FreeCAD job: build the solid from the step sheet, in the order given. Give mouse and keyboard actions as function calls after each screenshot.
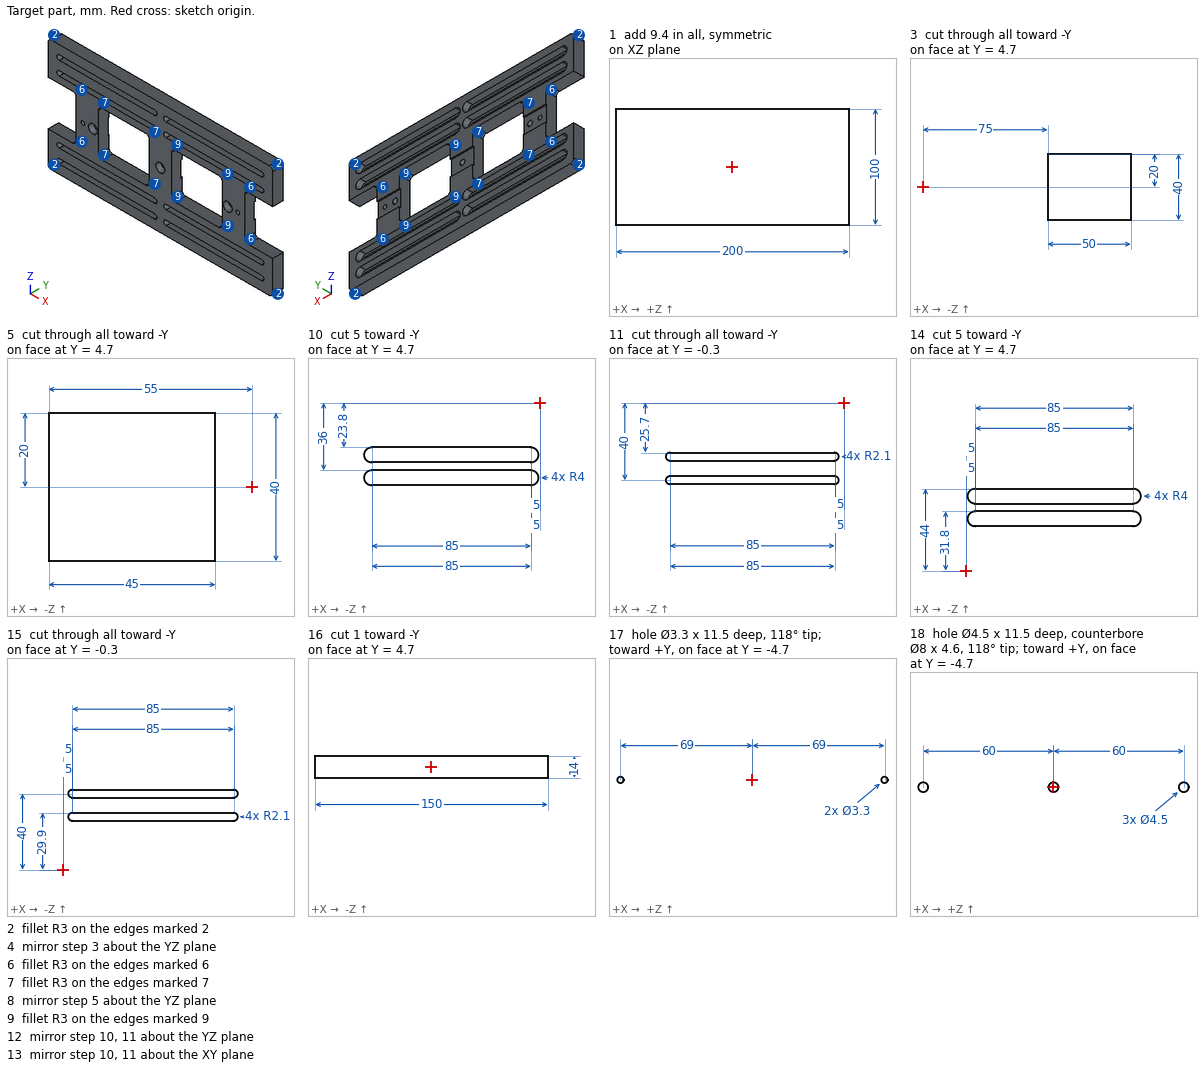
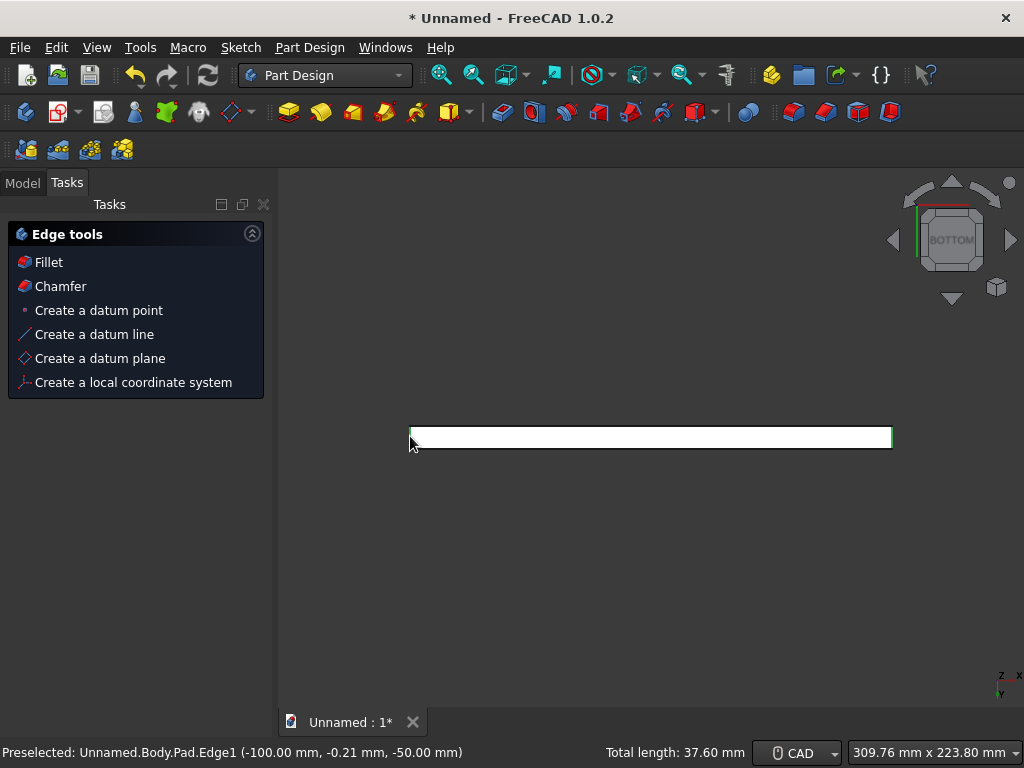
click(794, 112)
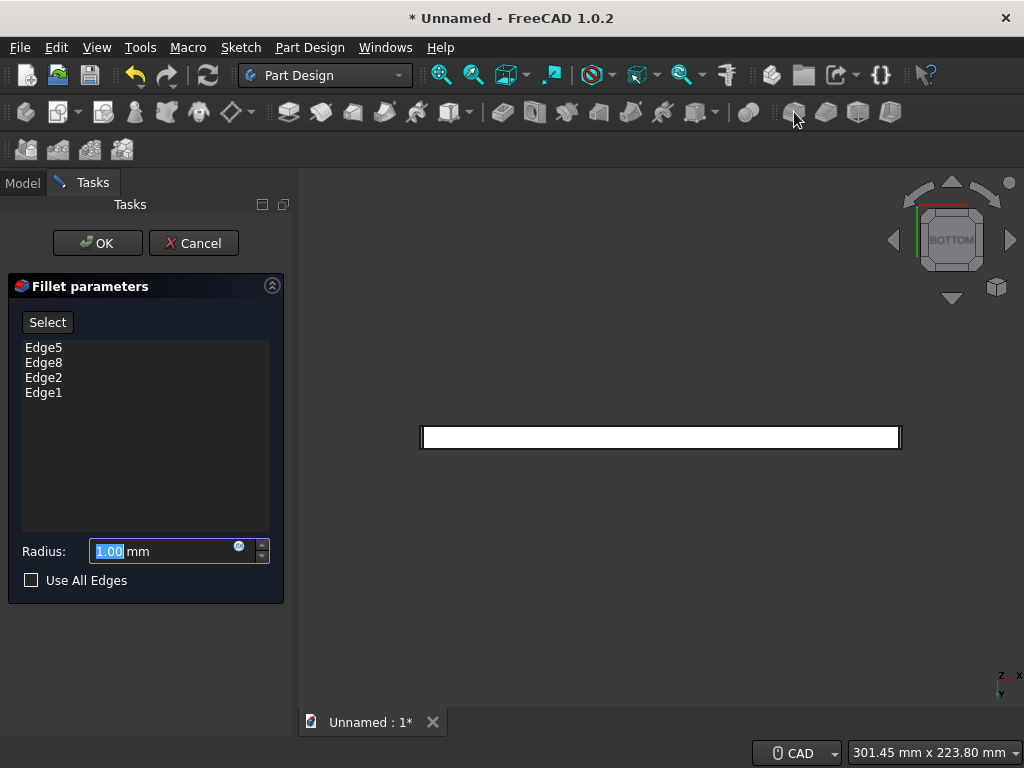
text(3)
key(Tab)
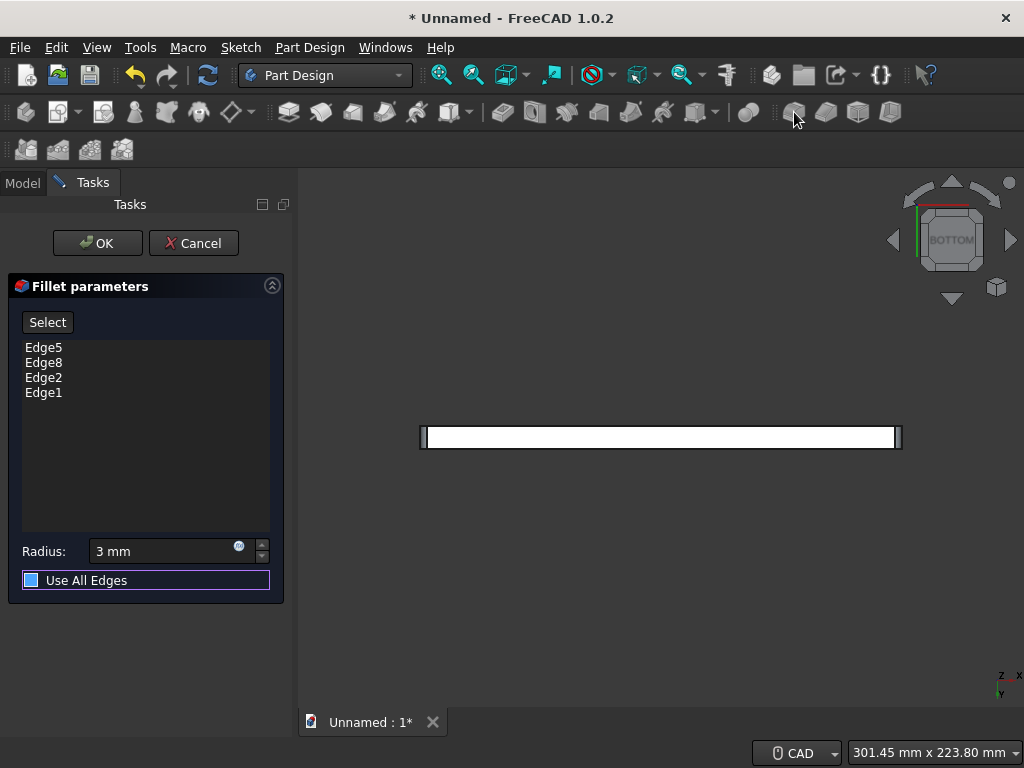
click(98, 243)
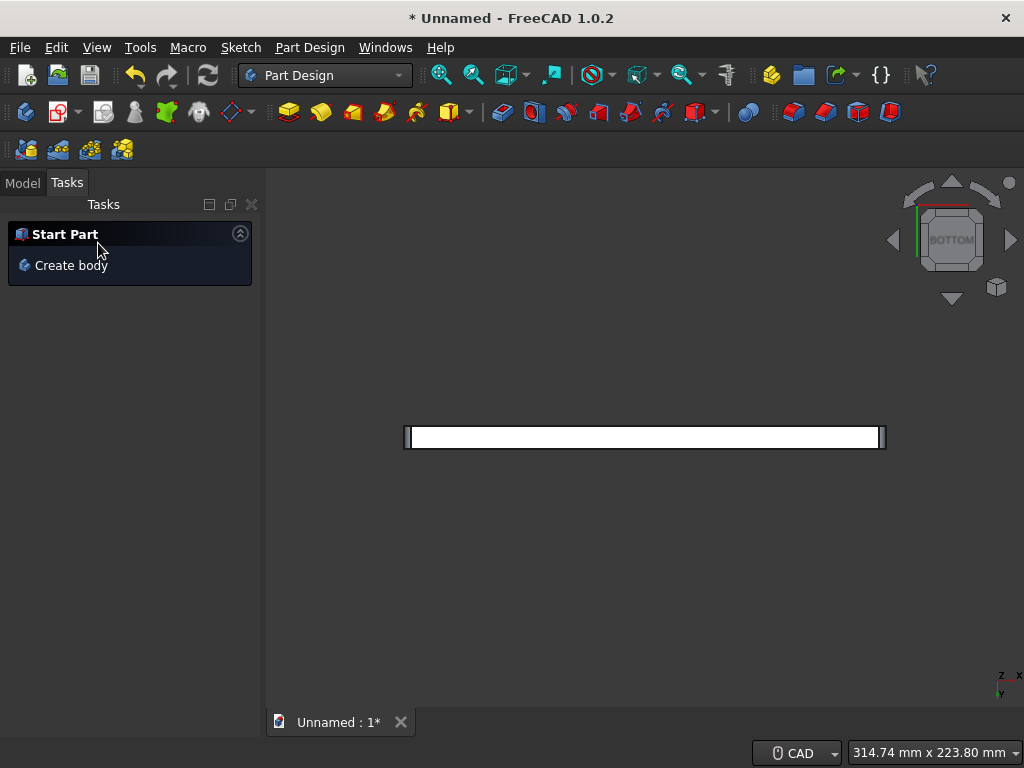
key(4)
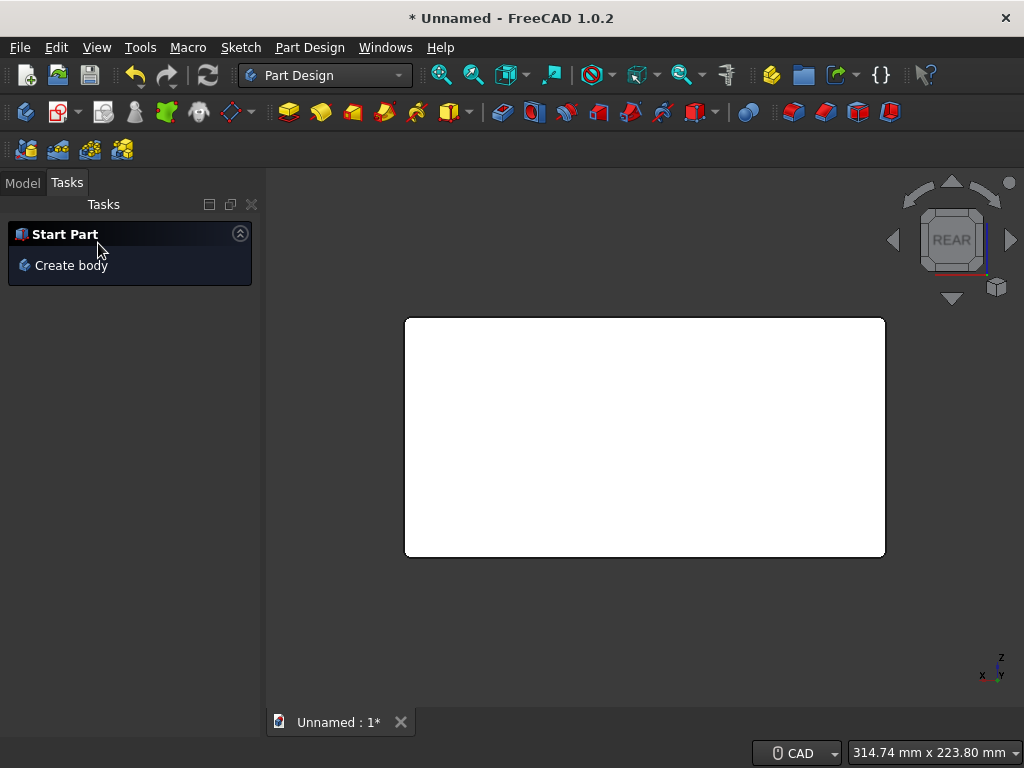
click(576, 437)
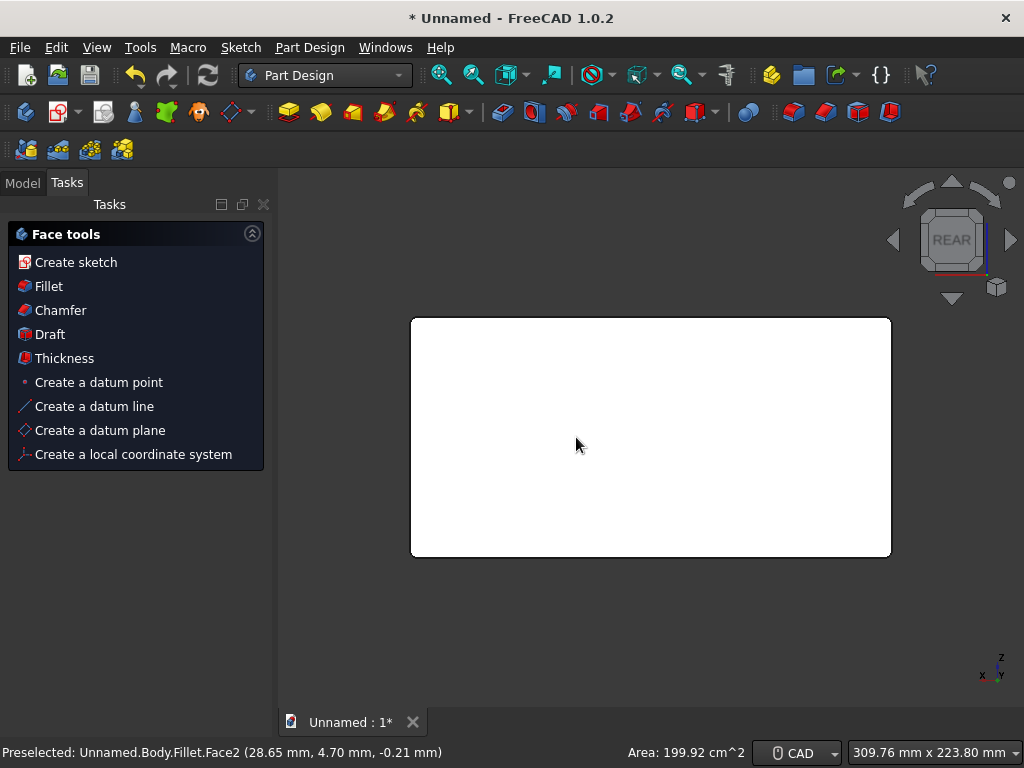
click(58, 112)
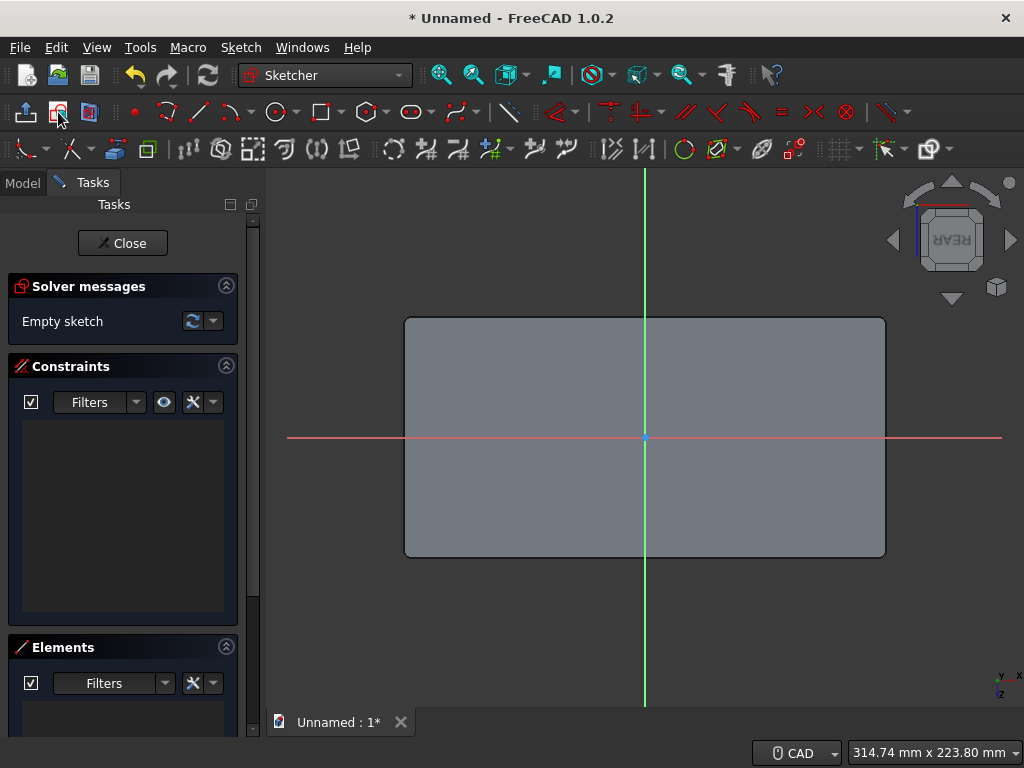
scroll(576, 438, down, 5)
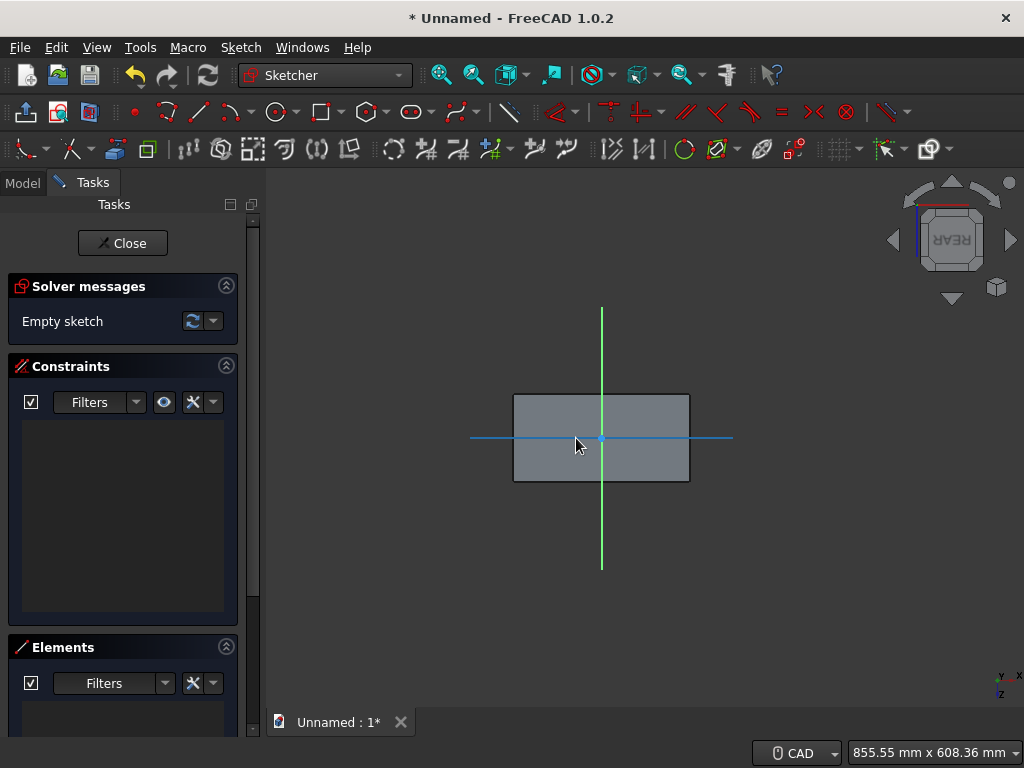
scroll(704, 438, up, 11)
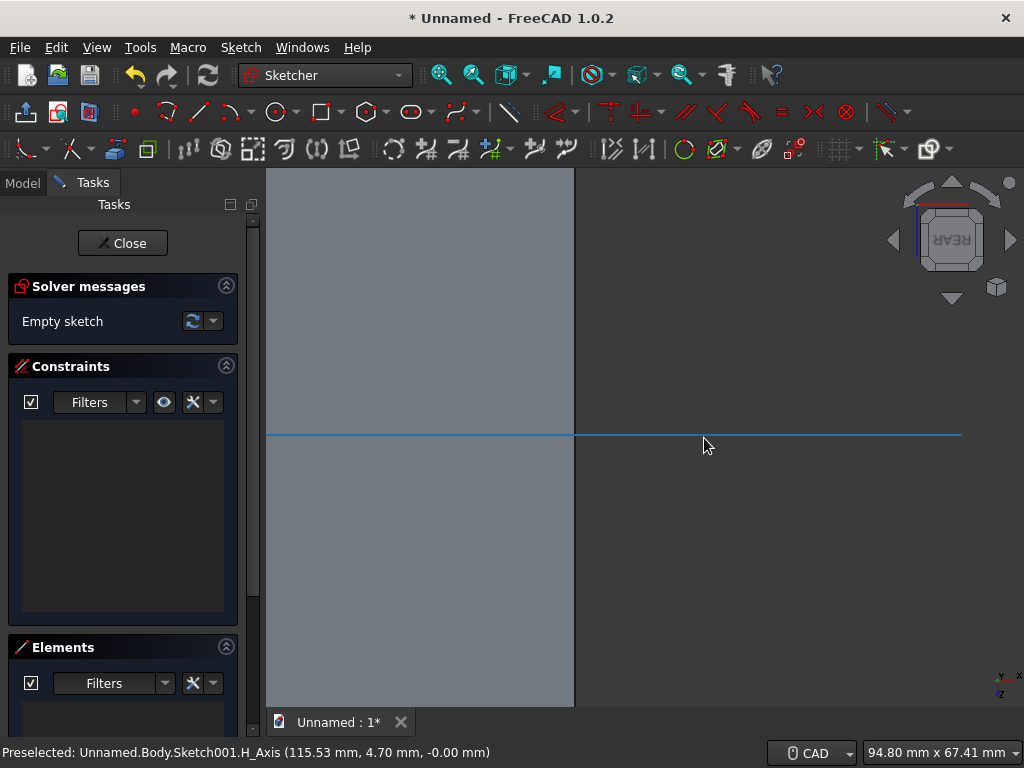
key(g)
key(r)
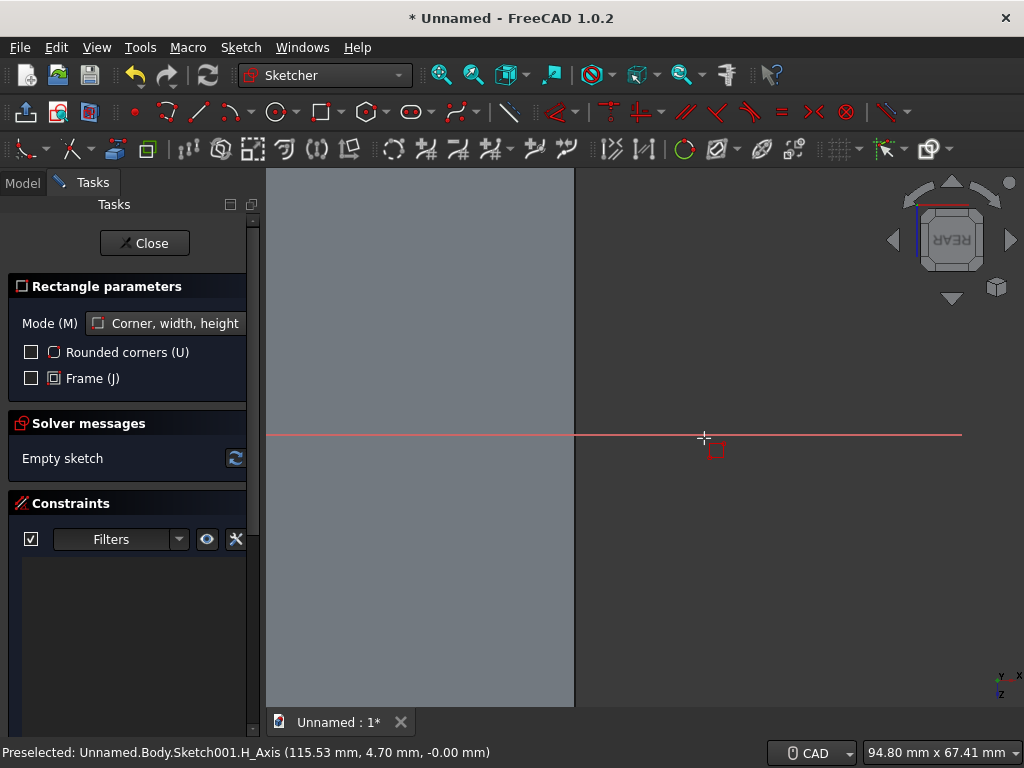
click(375, 275)
move(775, 595)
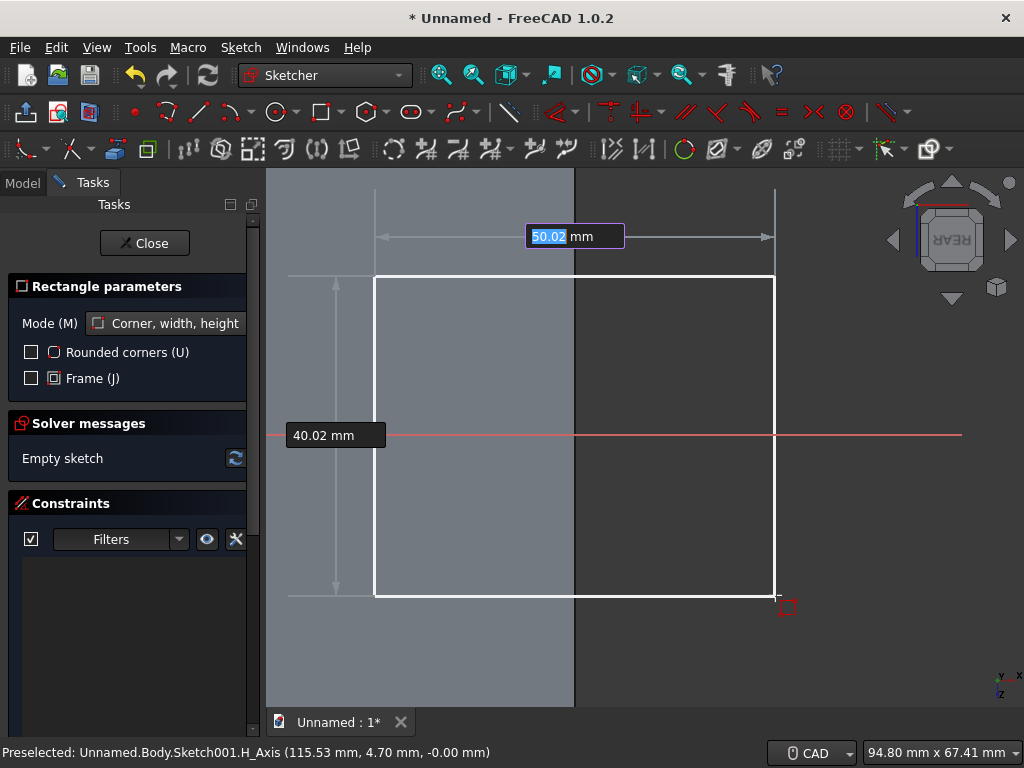
text(50)
key(Tab)
text(40)
key(Return)
key(Escape)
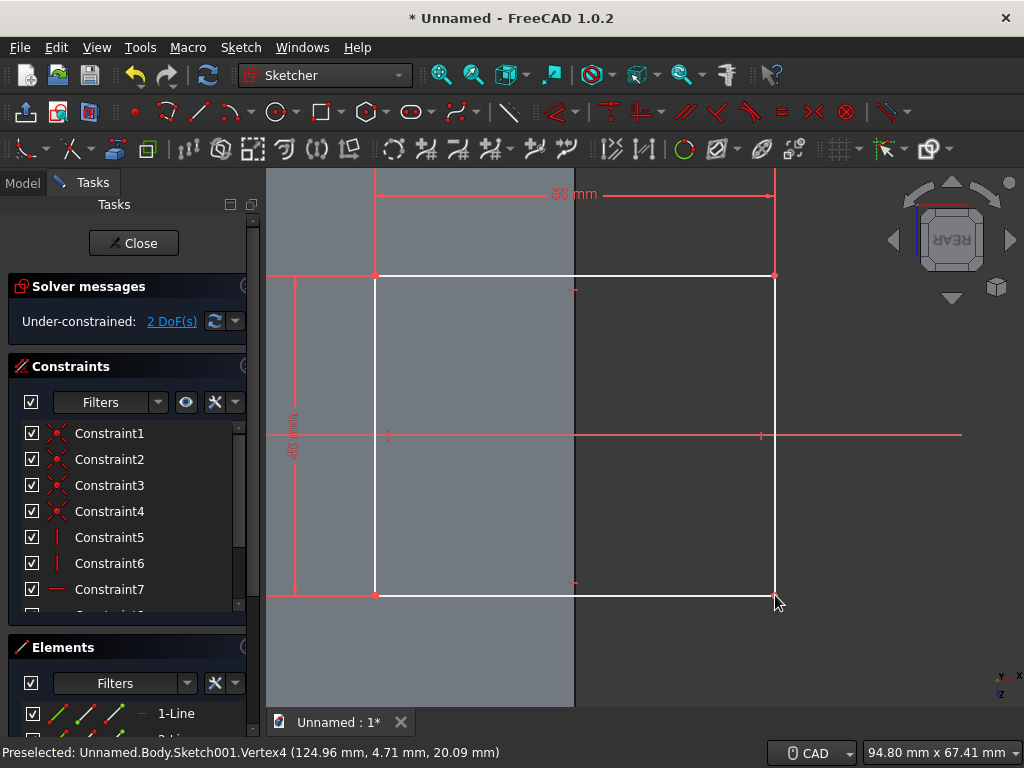
key(d)